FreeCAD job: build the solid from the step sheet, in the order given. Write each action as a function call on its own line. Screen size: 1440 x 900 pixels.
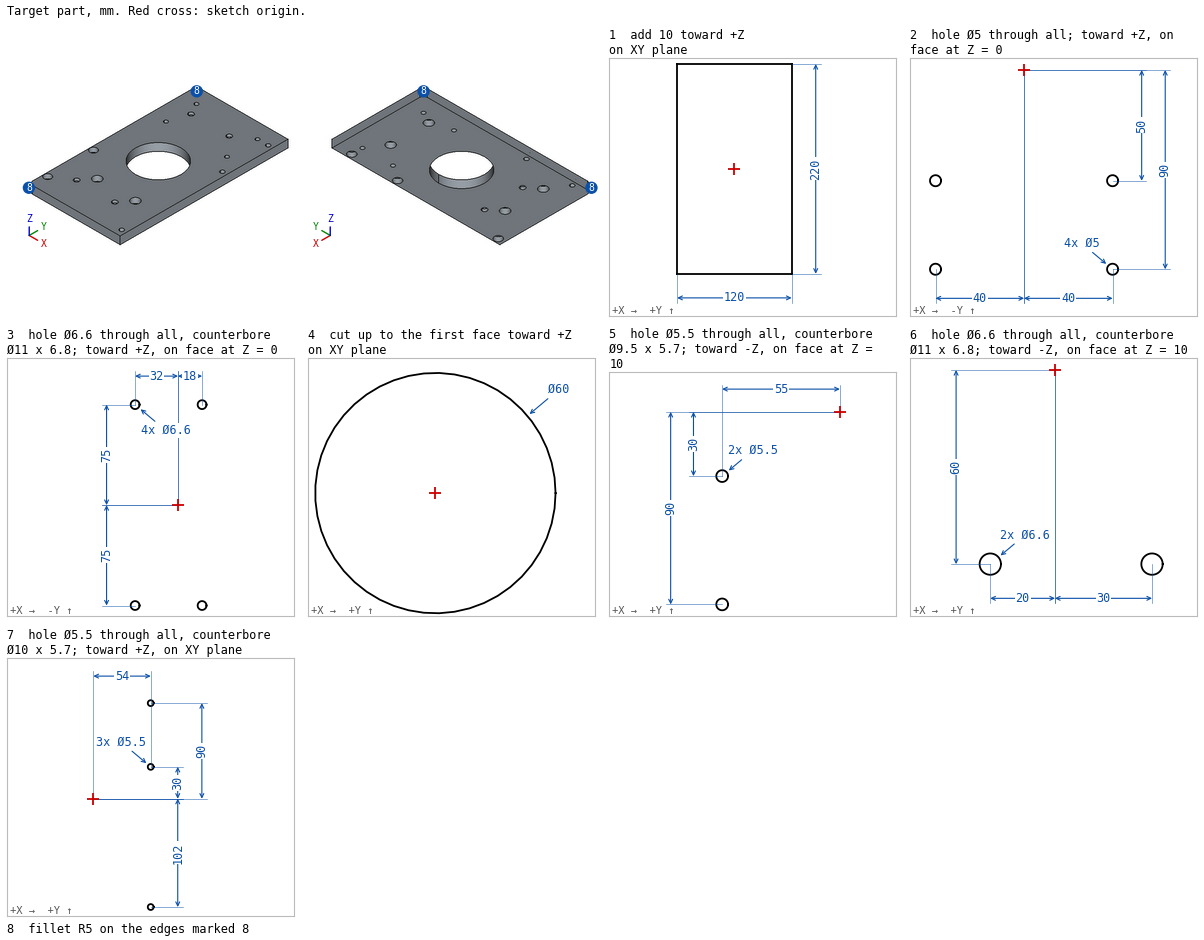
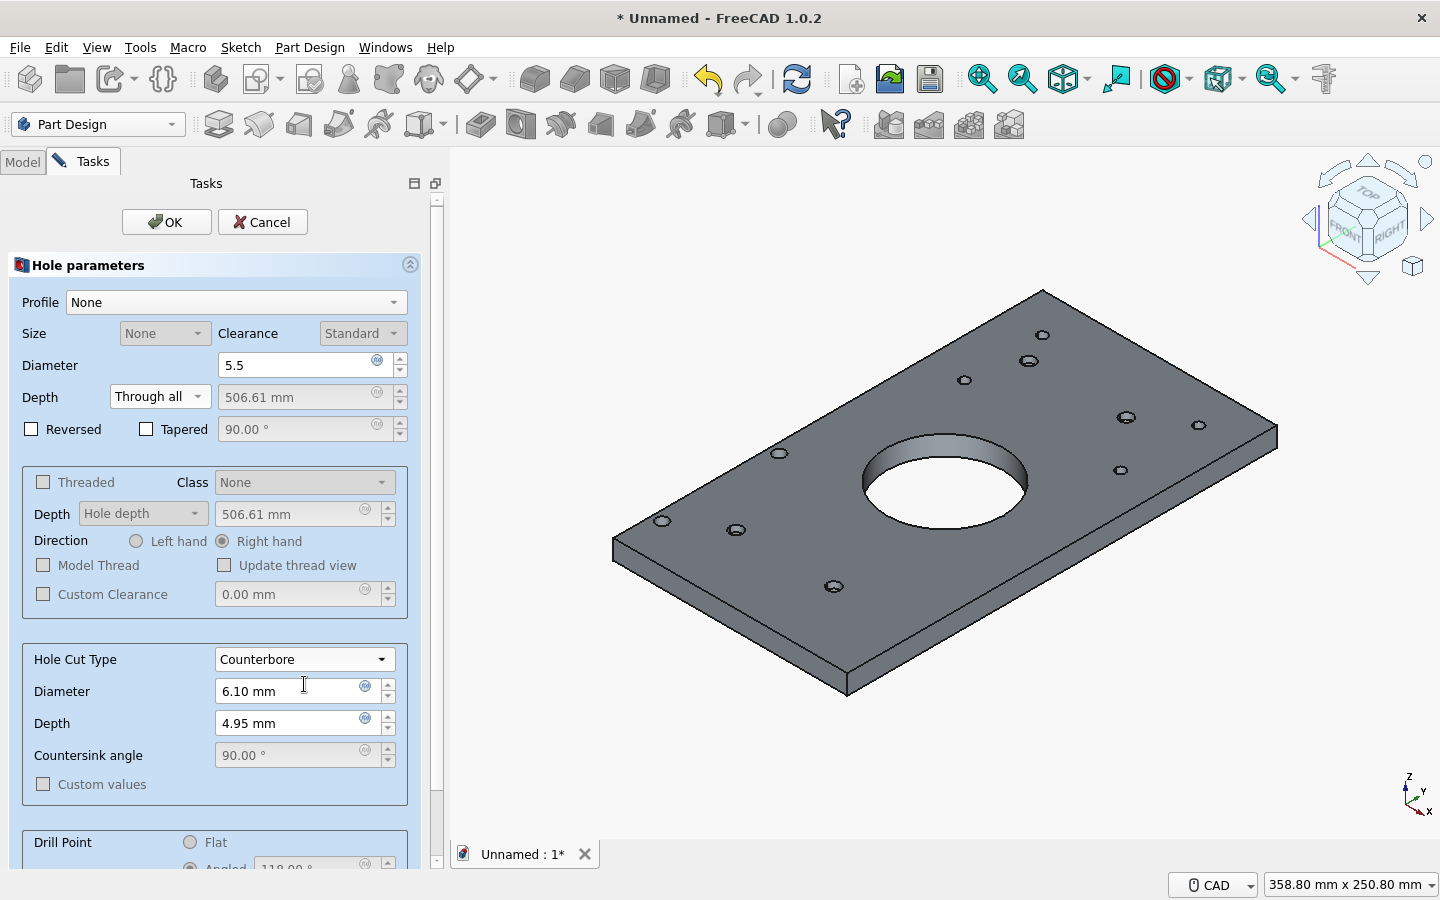
triple_click(298, 691)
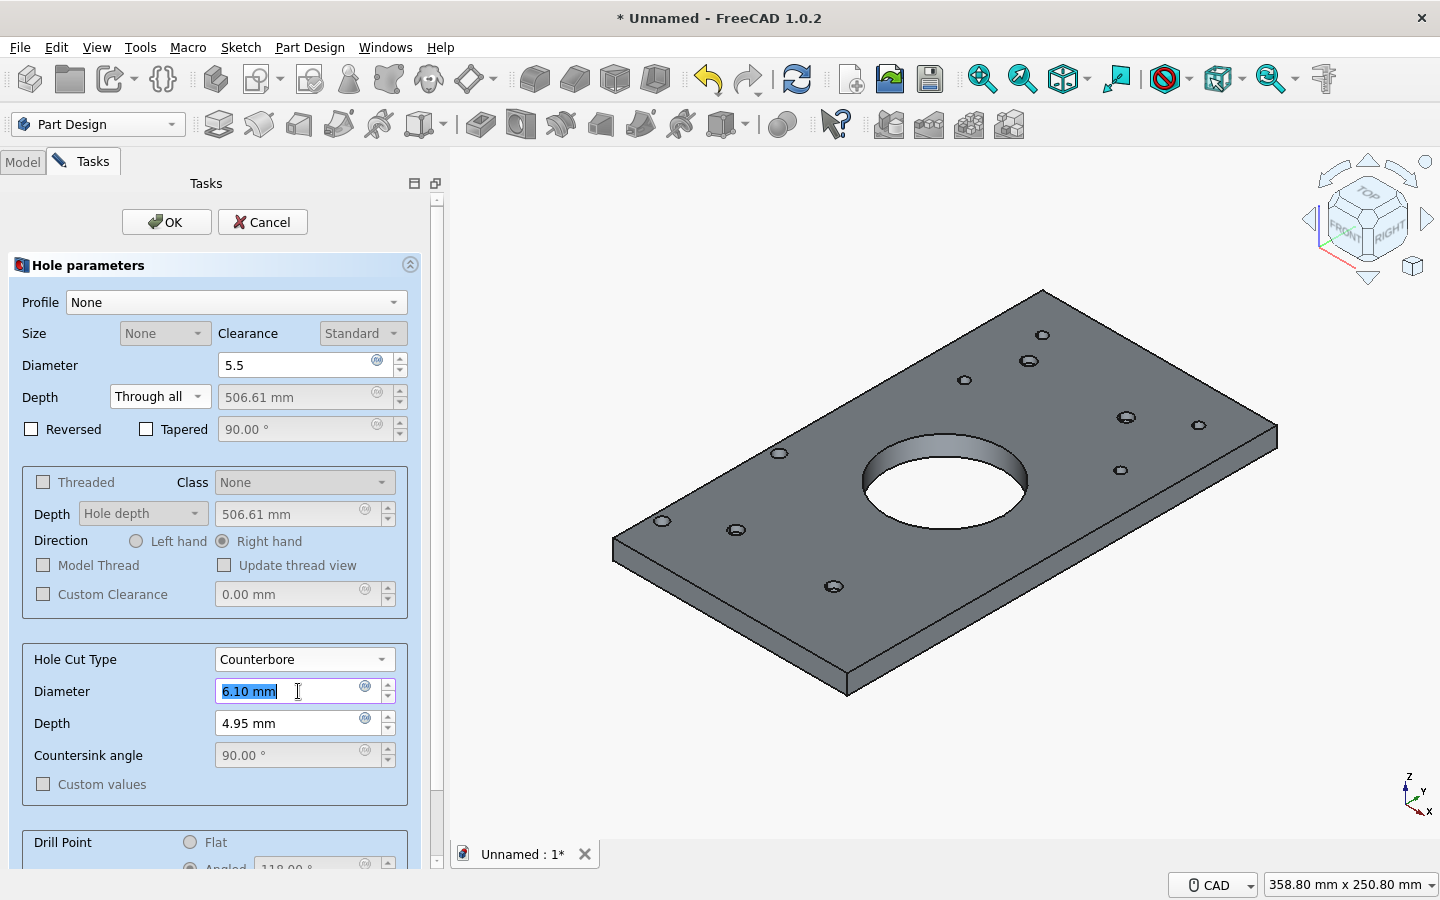
text(9.5)
key(Tab)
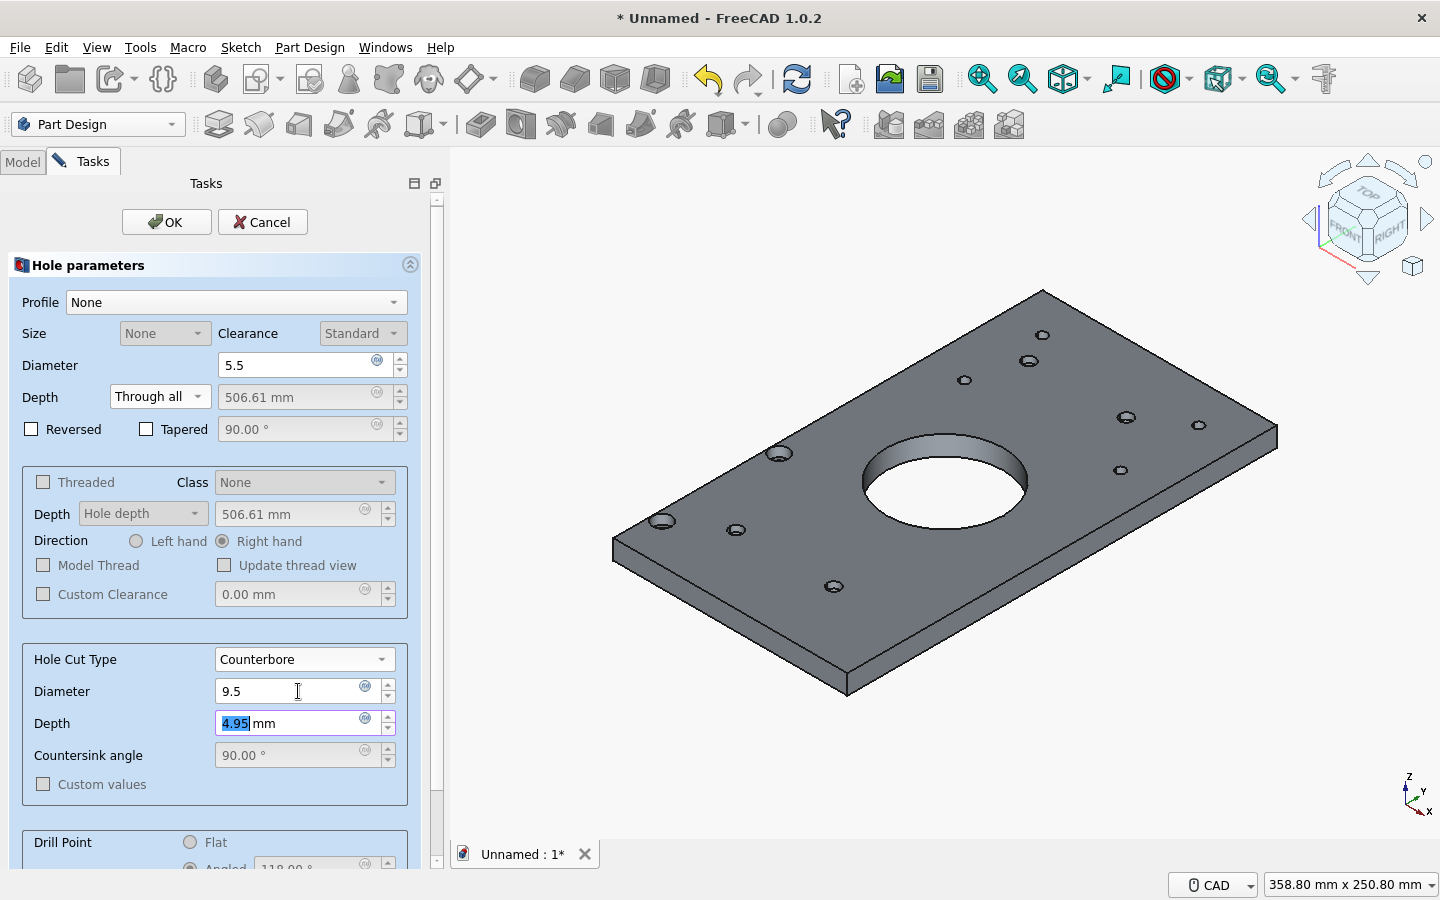
text(5.7)
key(Tab)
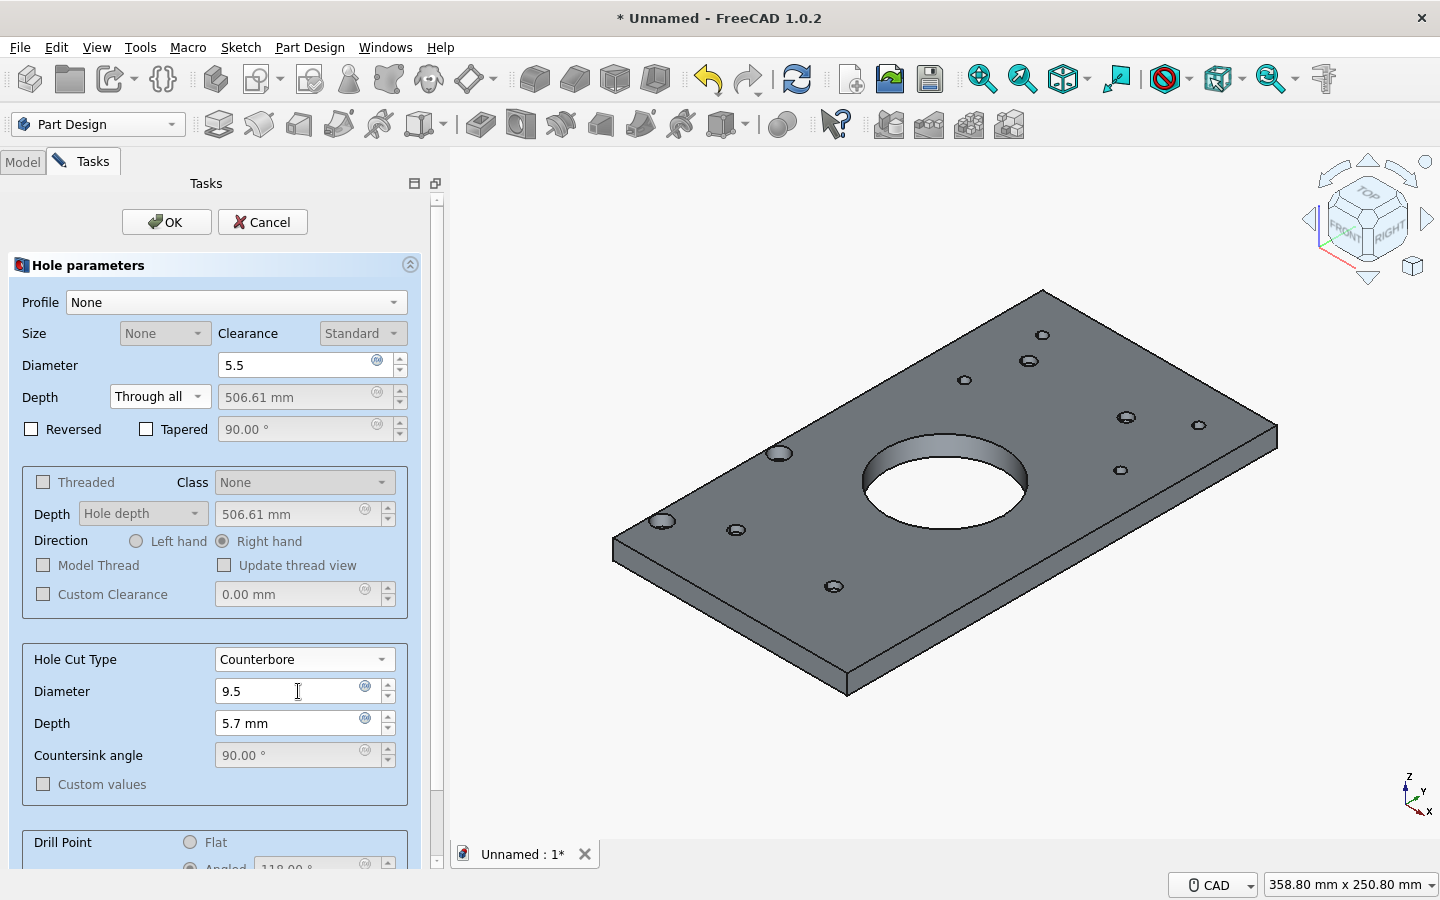
click(167, 222)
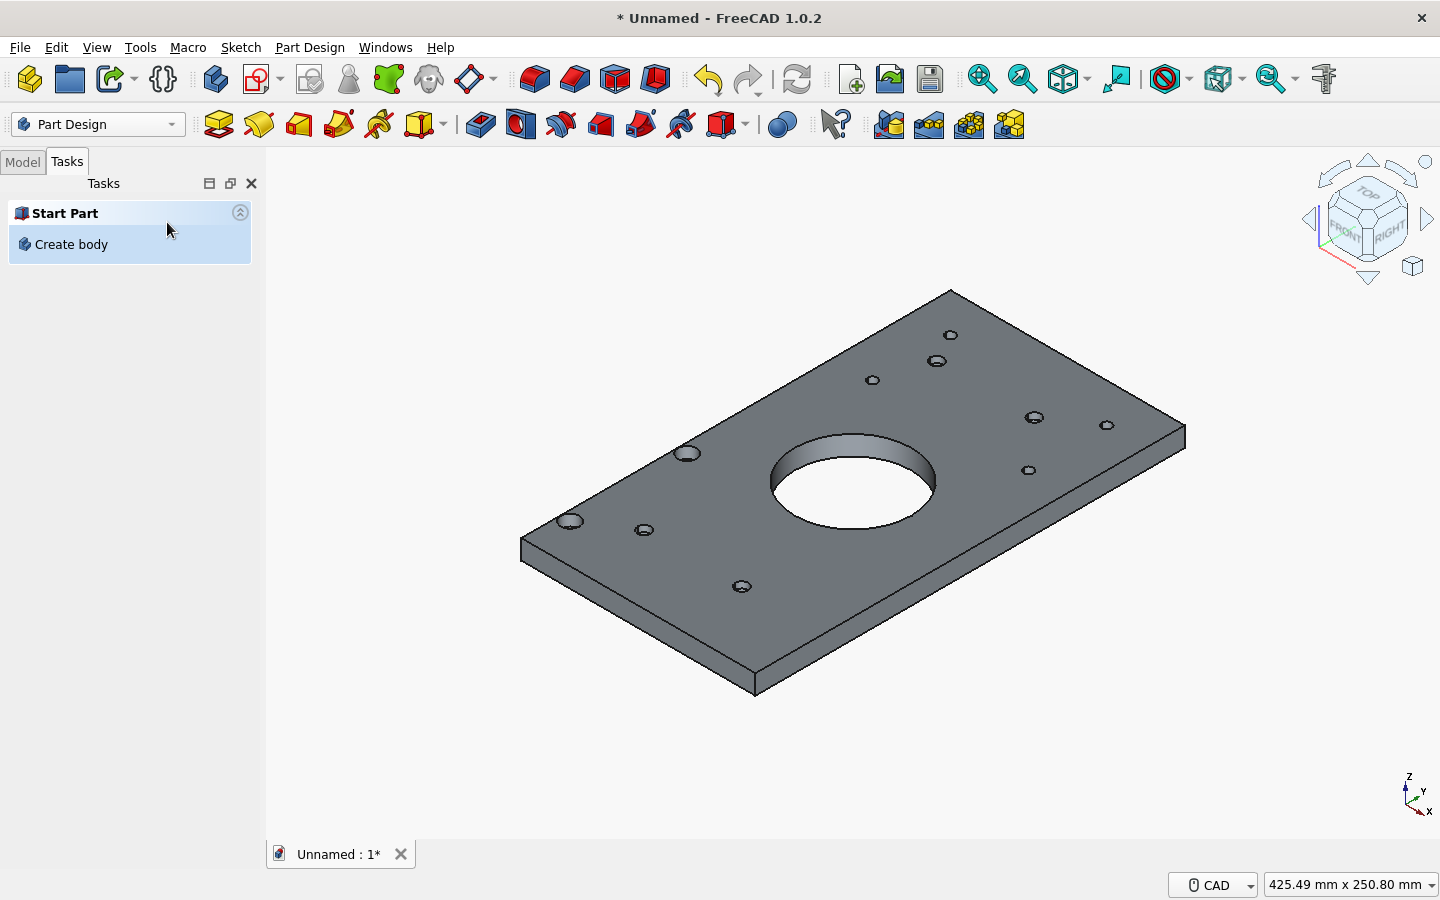
click(730, 552)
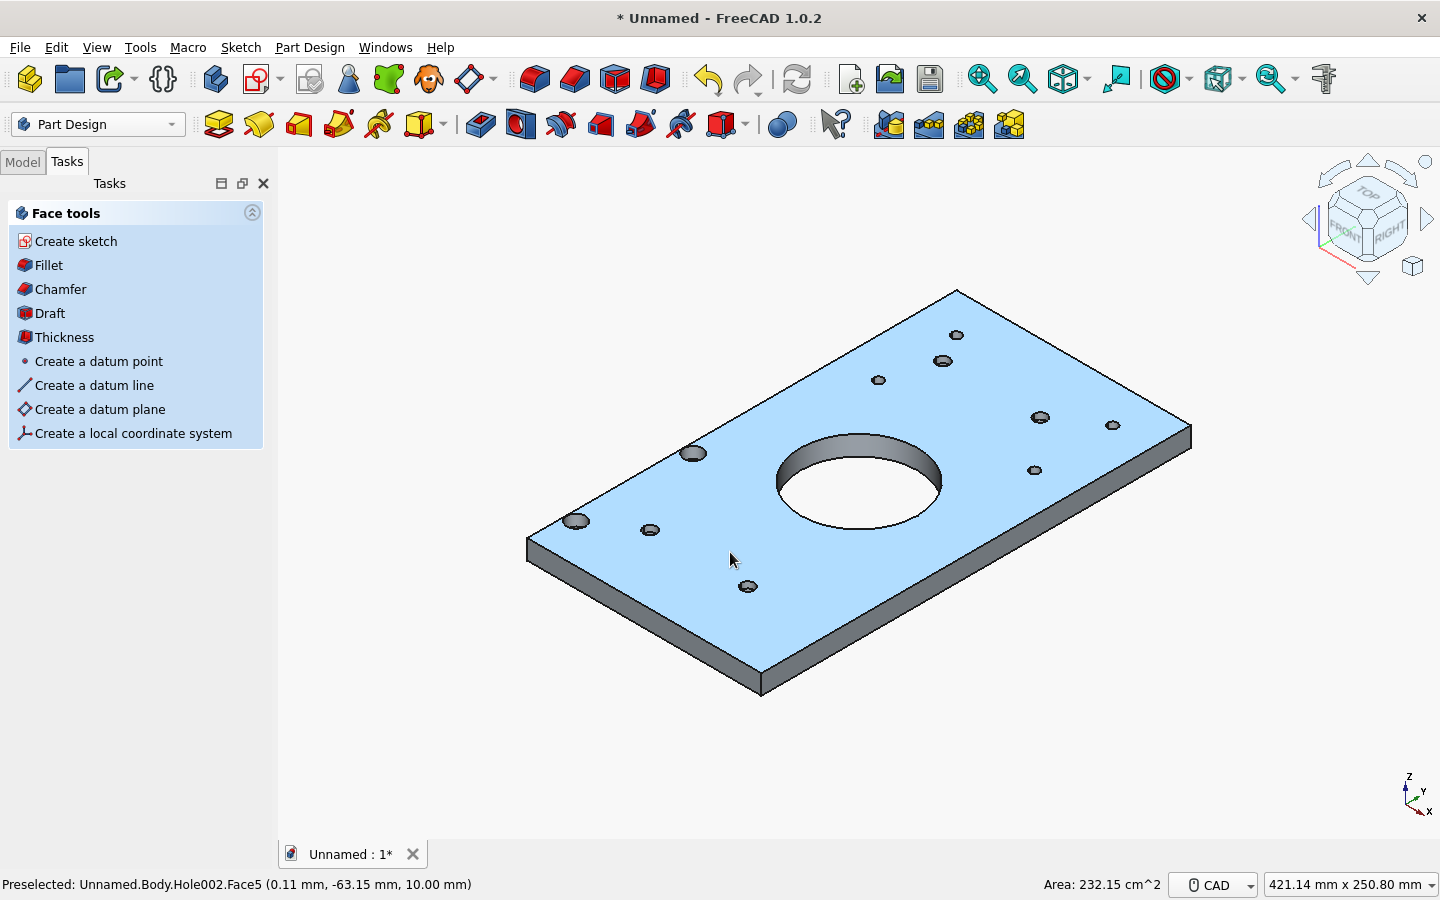
click(256, 80)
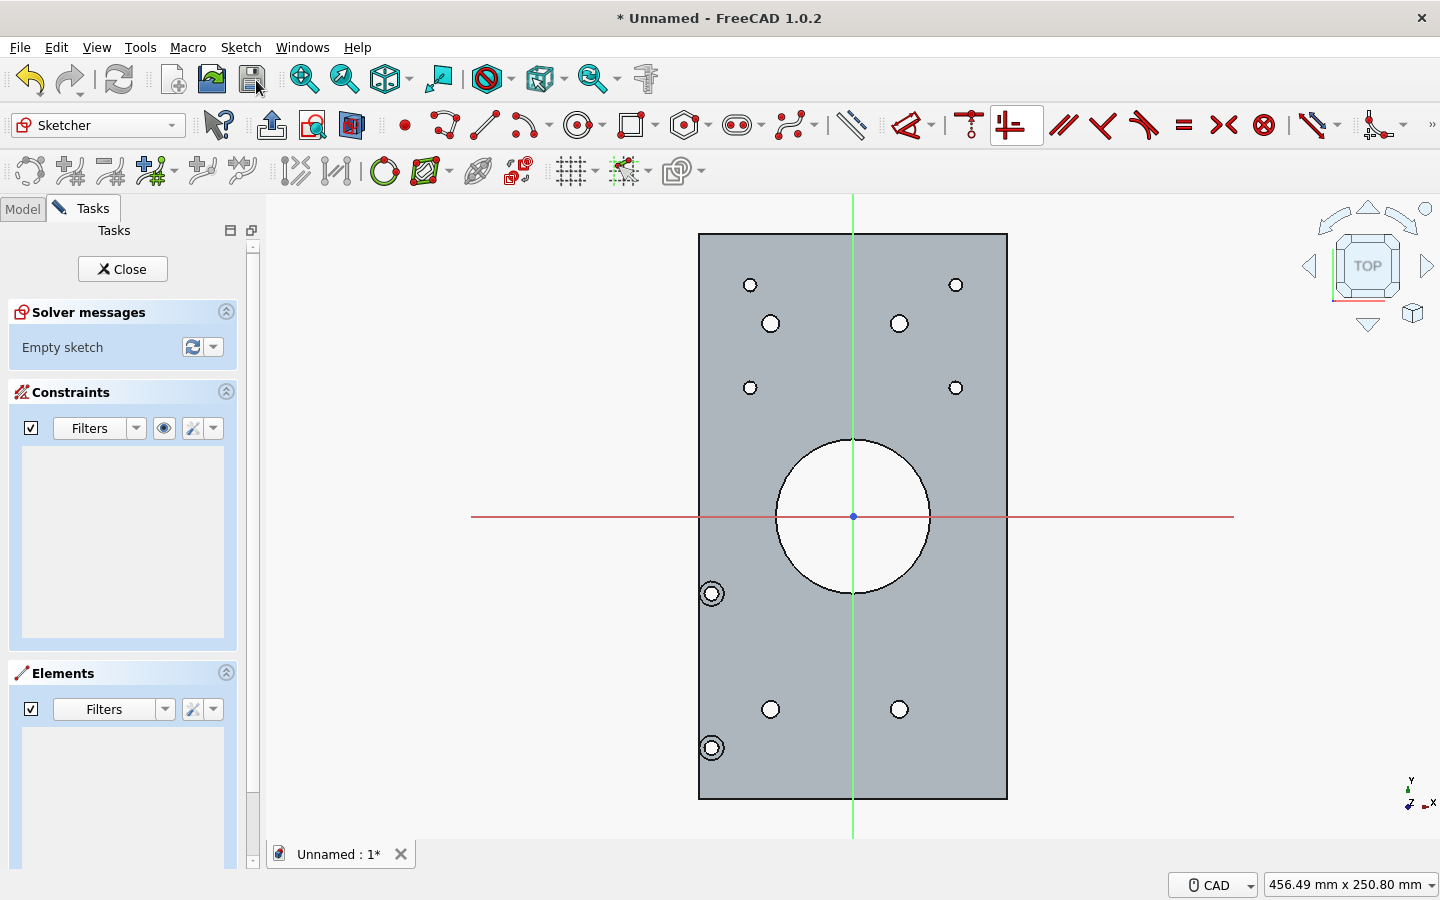
scroll(913, 645, up, 5)